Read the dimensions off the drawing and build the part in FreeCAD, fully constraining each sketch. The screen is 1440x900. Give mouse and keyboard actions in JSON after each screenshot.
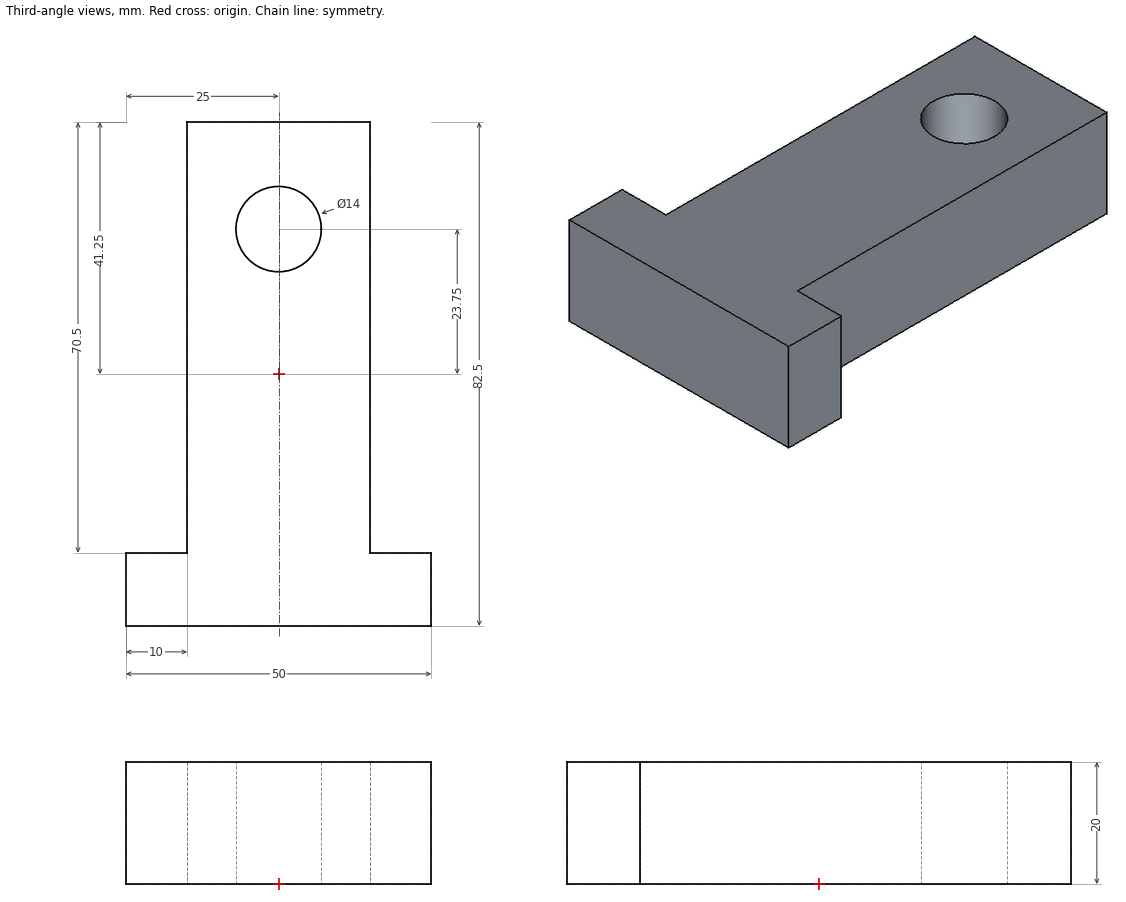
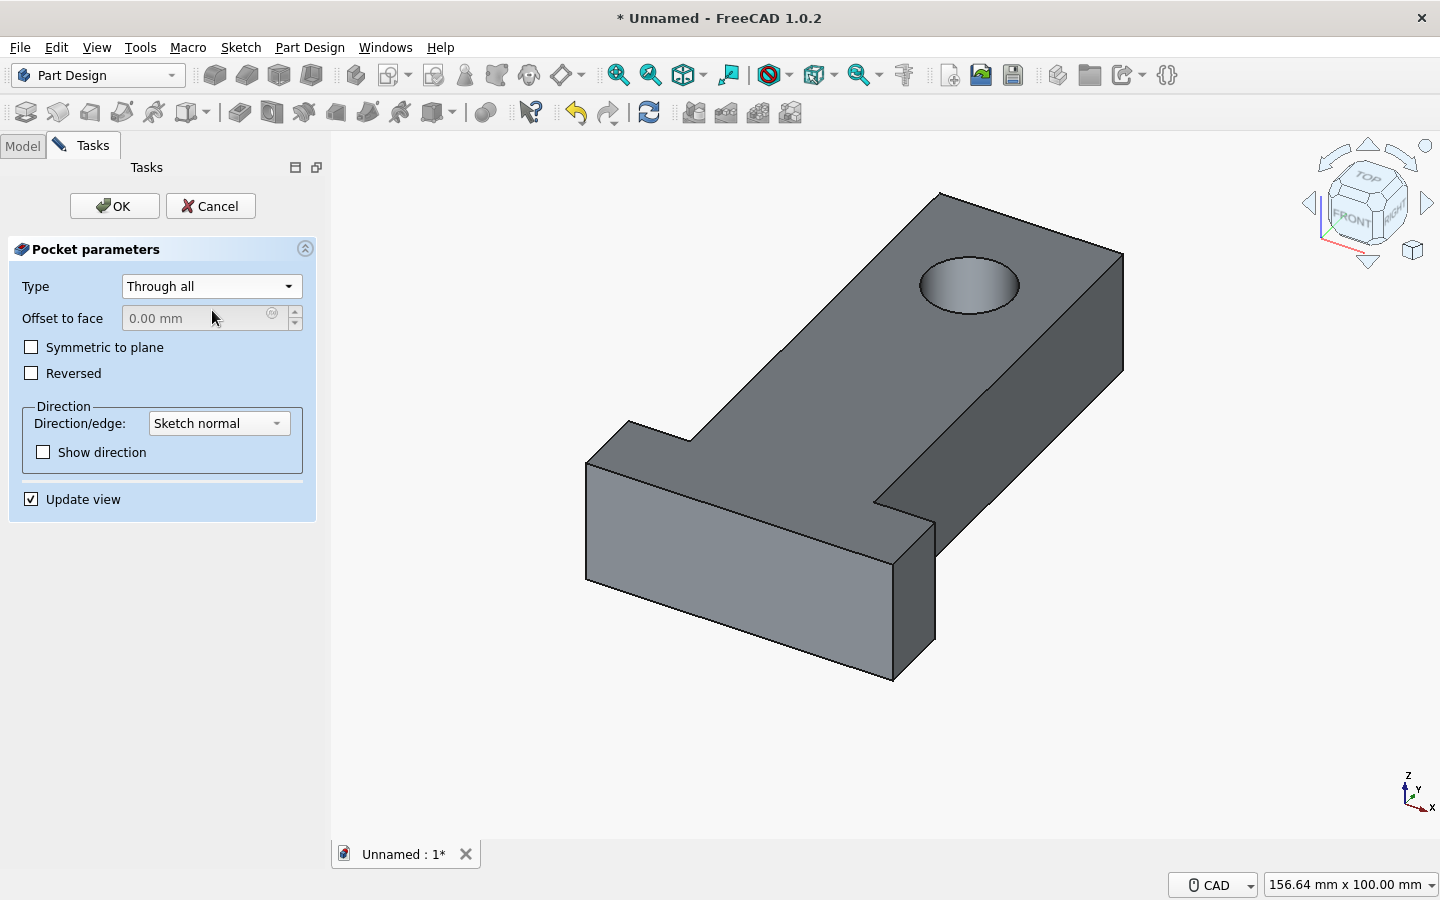
{"action": "left_click", "coordinate": [115, 206]}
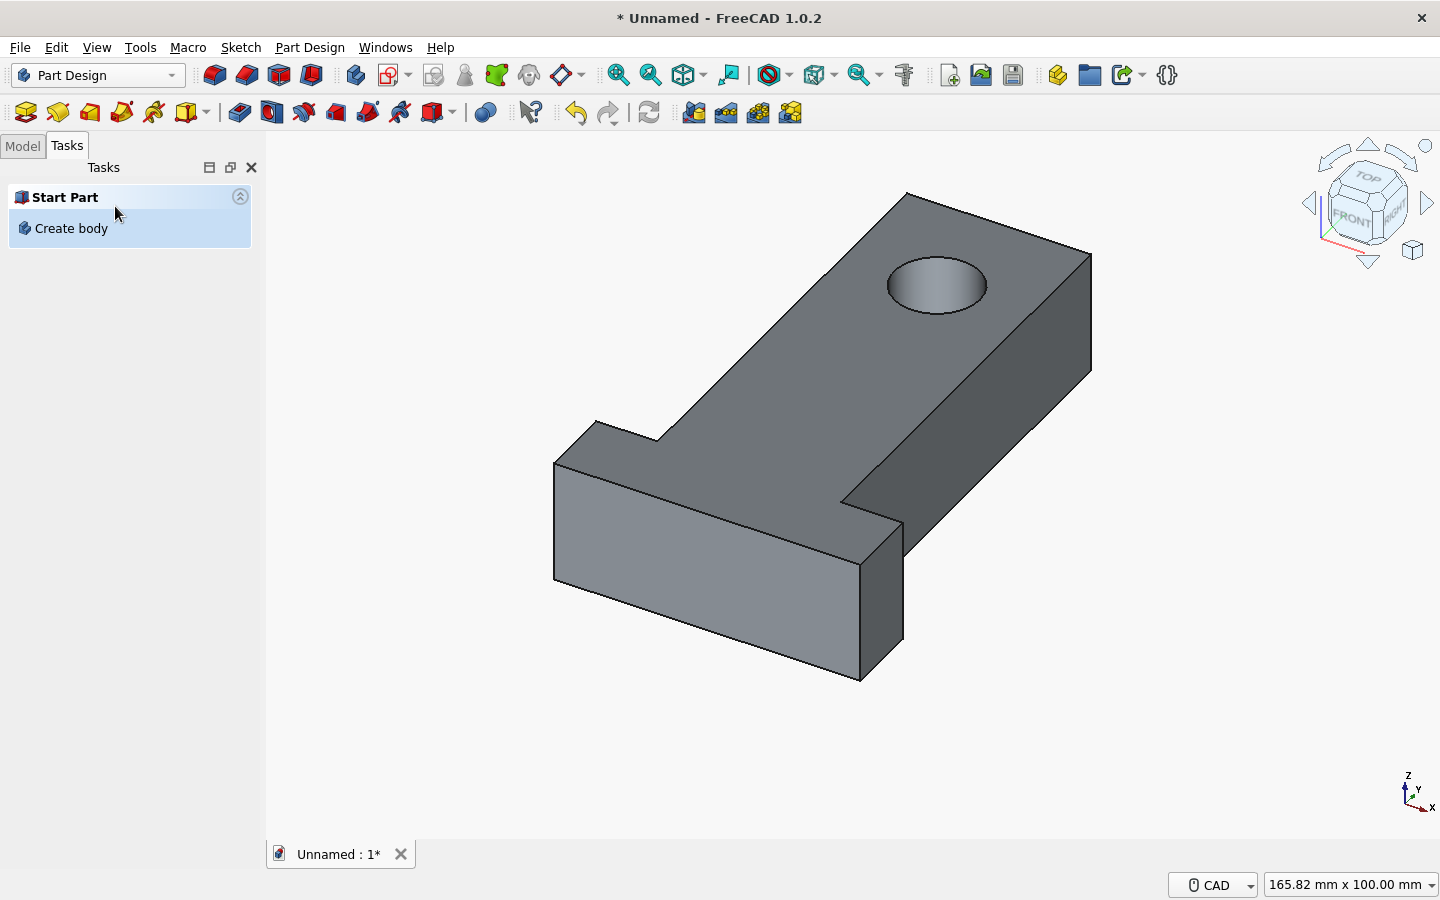
{"action": "key", "text": "0"}